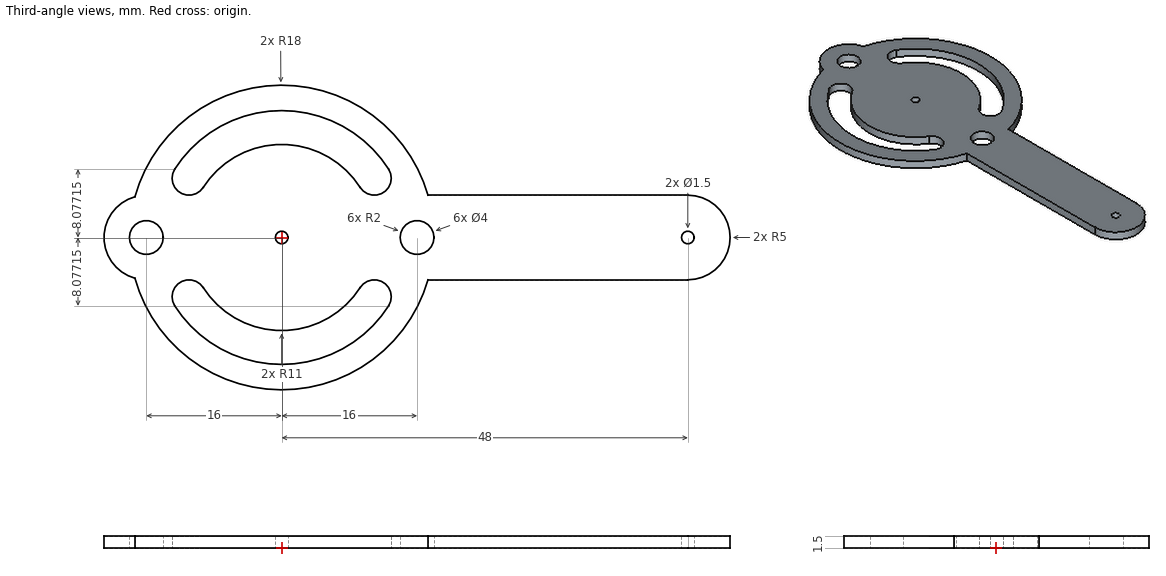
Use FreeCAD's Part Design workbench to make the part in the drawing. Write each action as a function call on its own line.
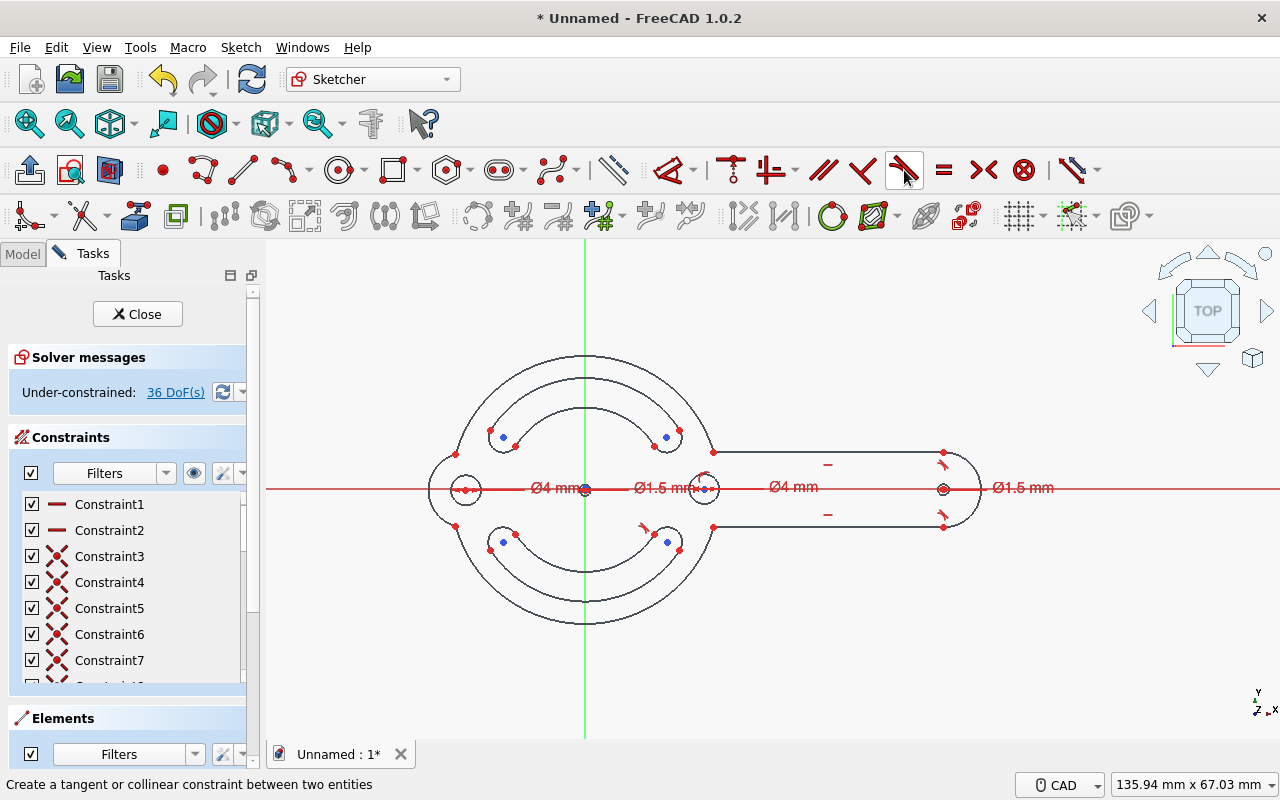
click(553, 565)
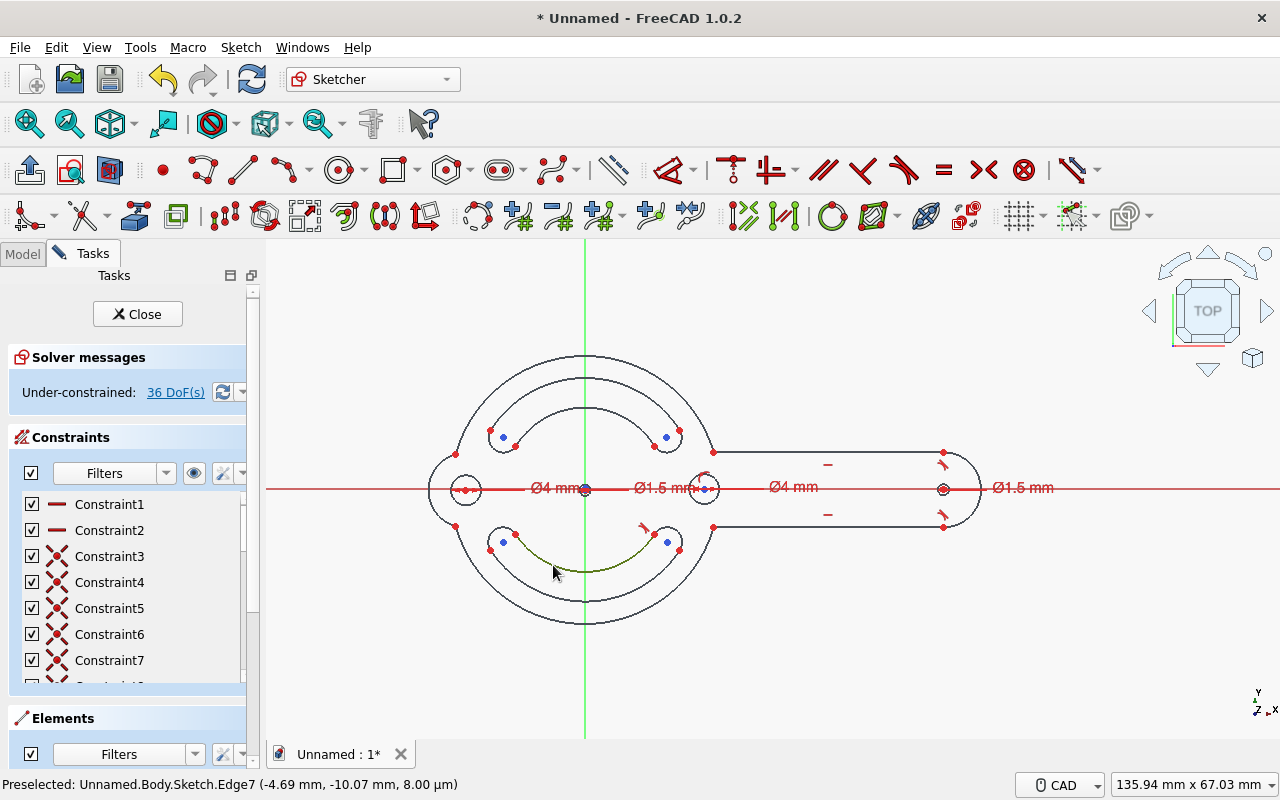
click(504, 527)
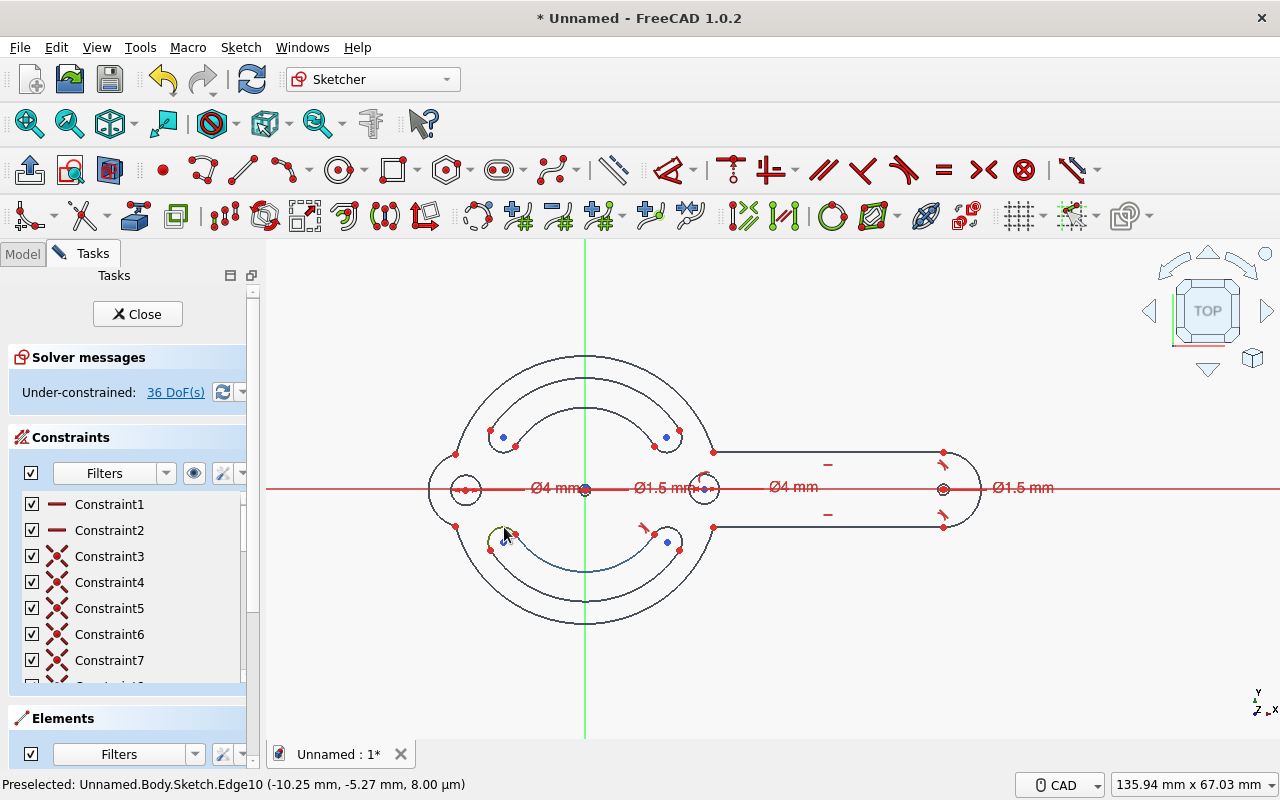
click(904, 170)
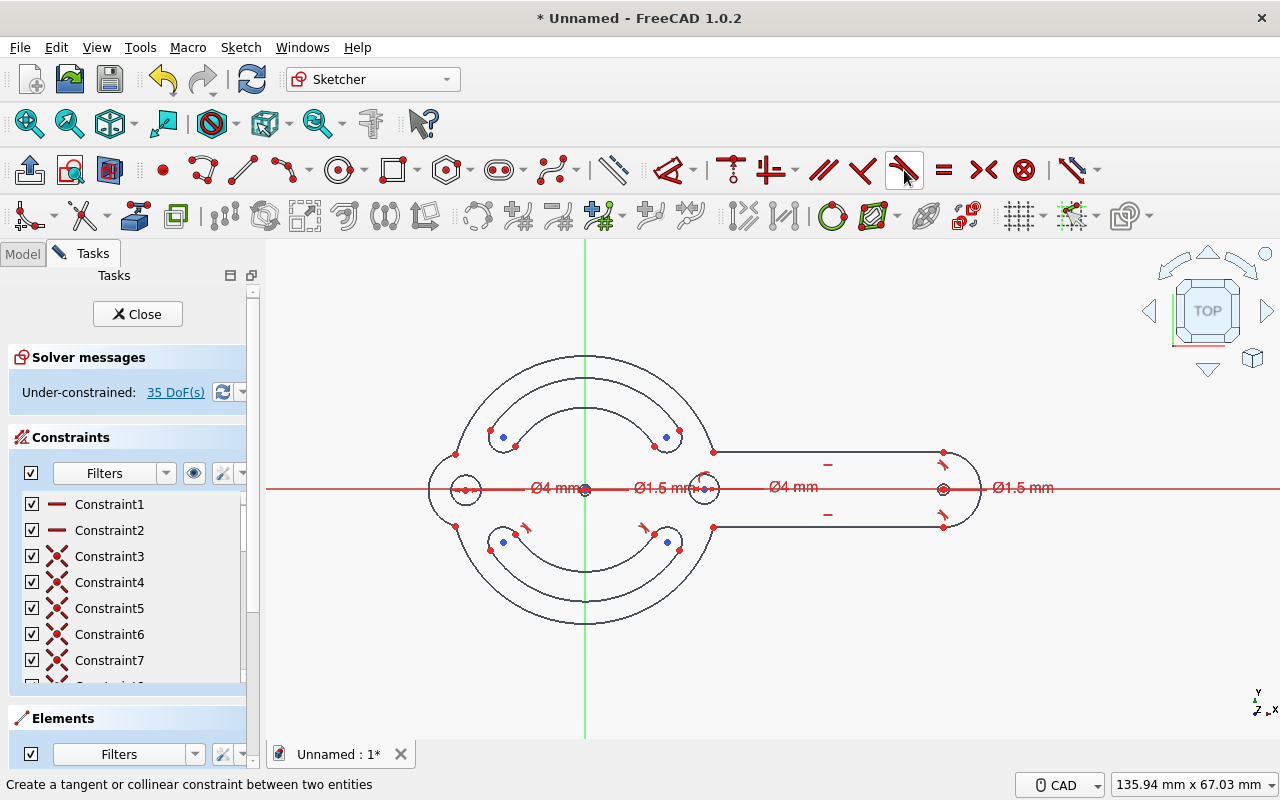
click(681, 537)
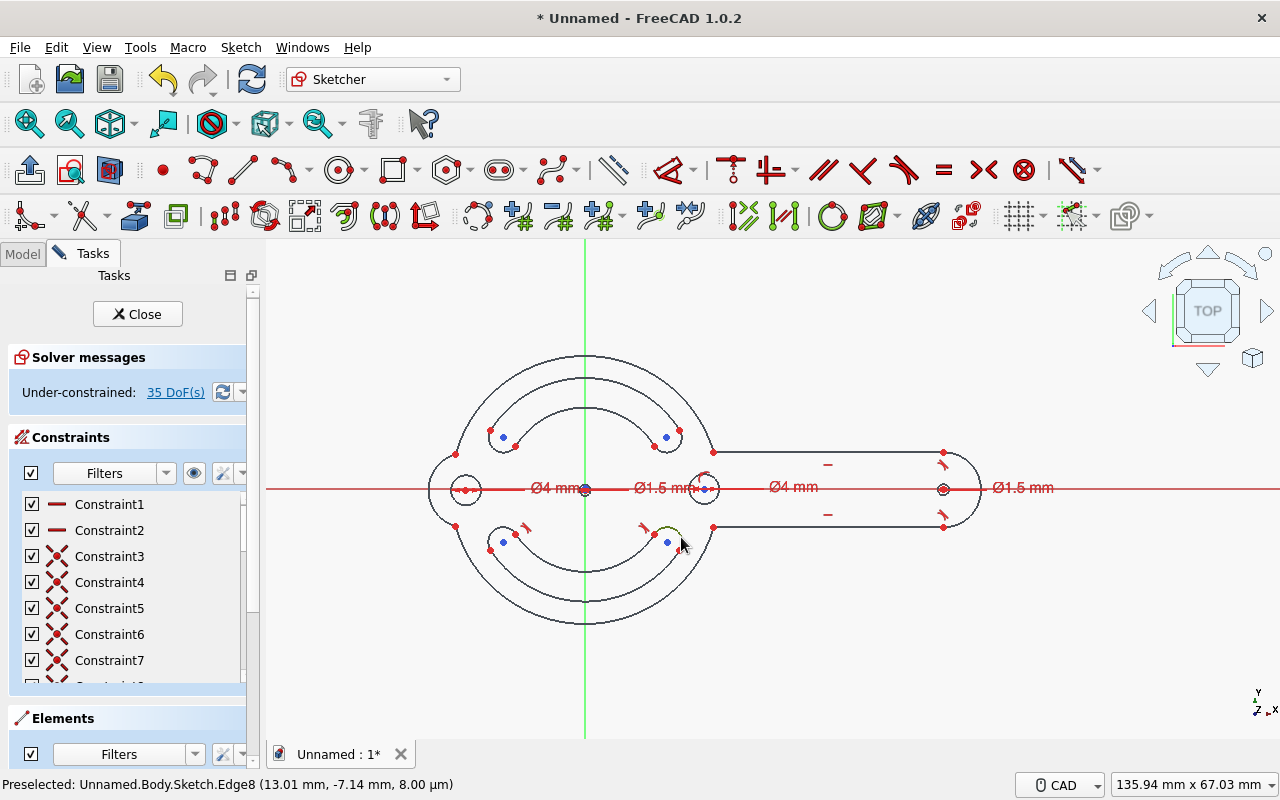
click(542, 593)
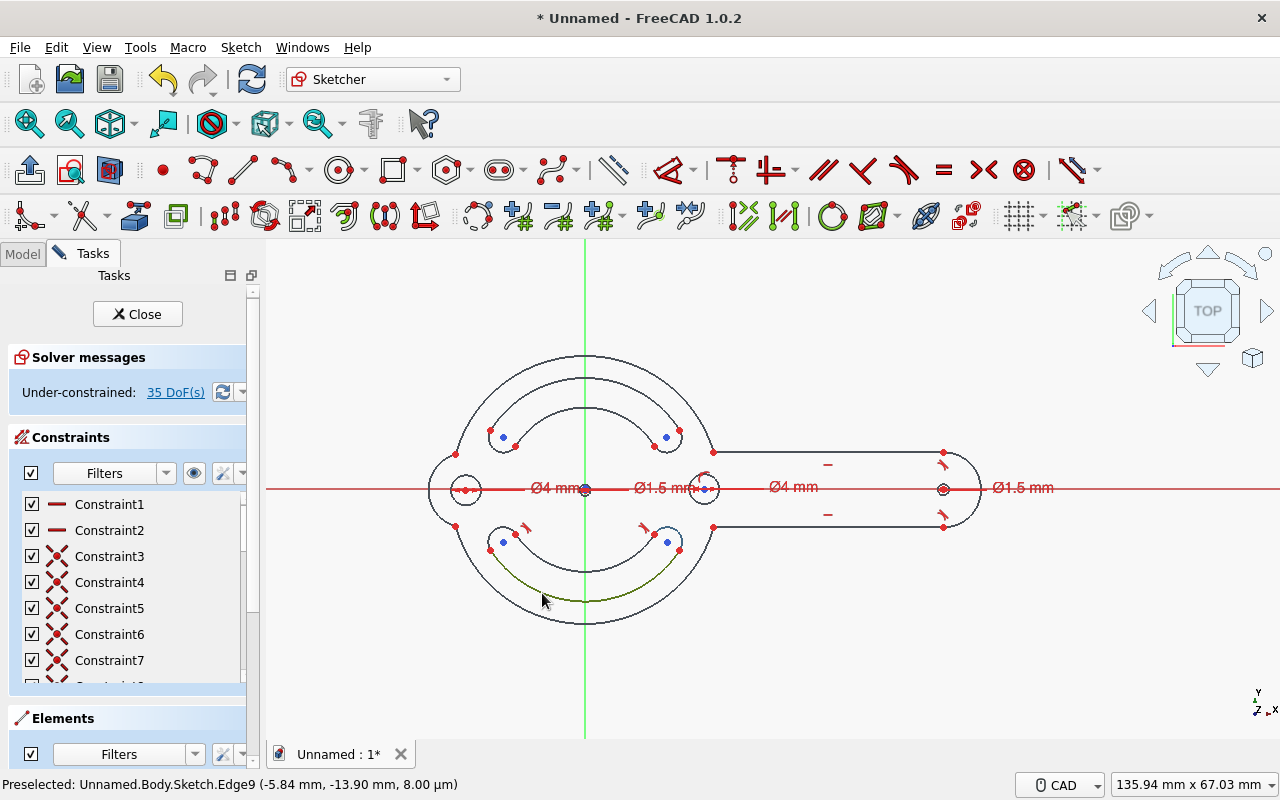
click(904, 170)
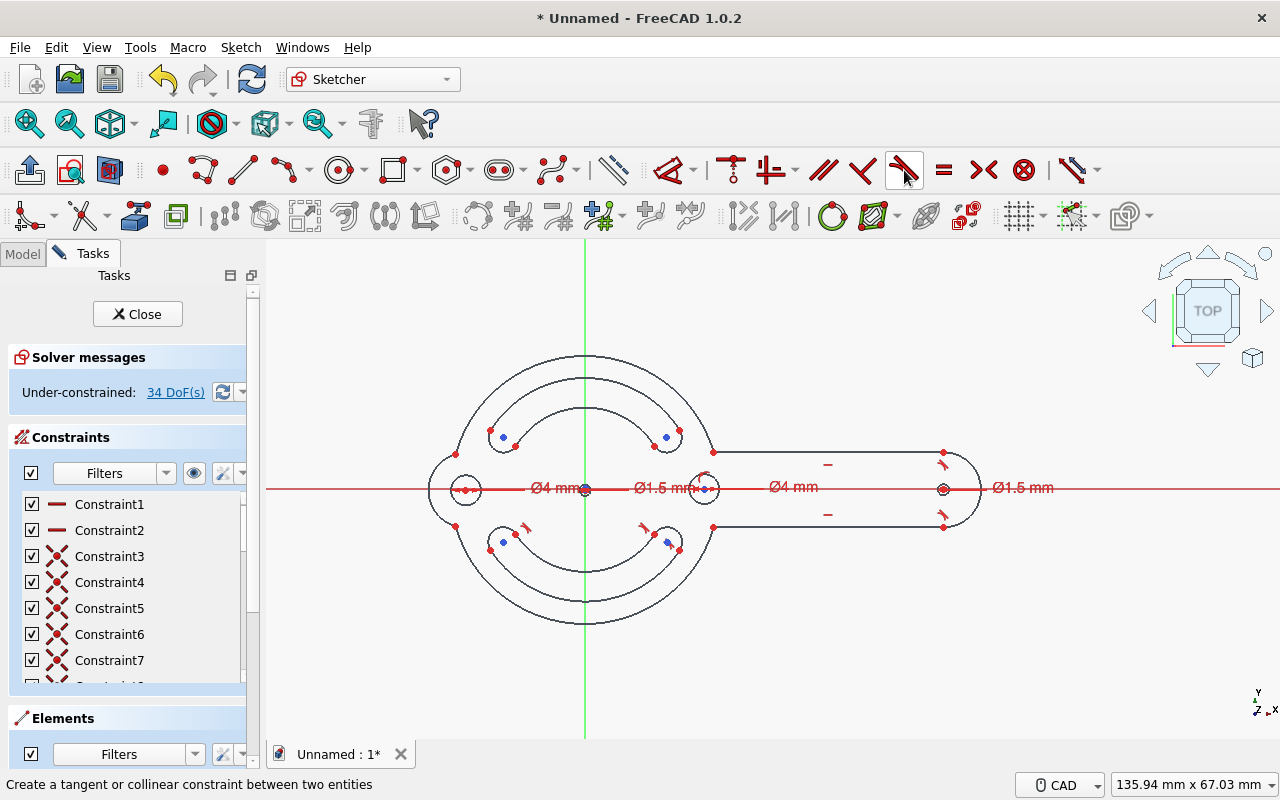
click(542, 593)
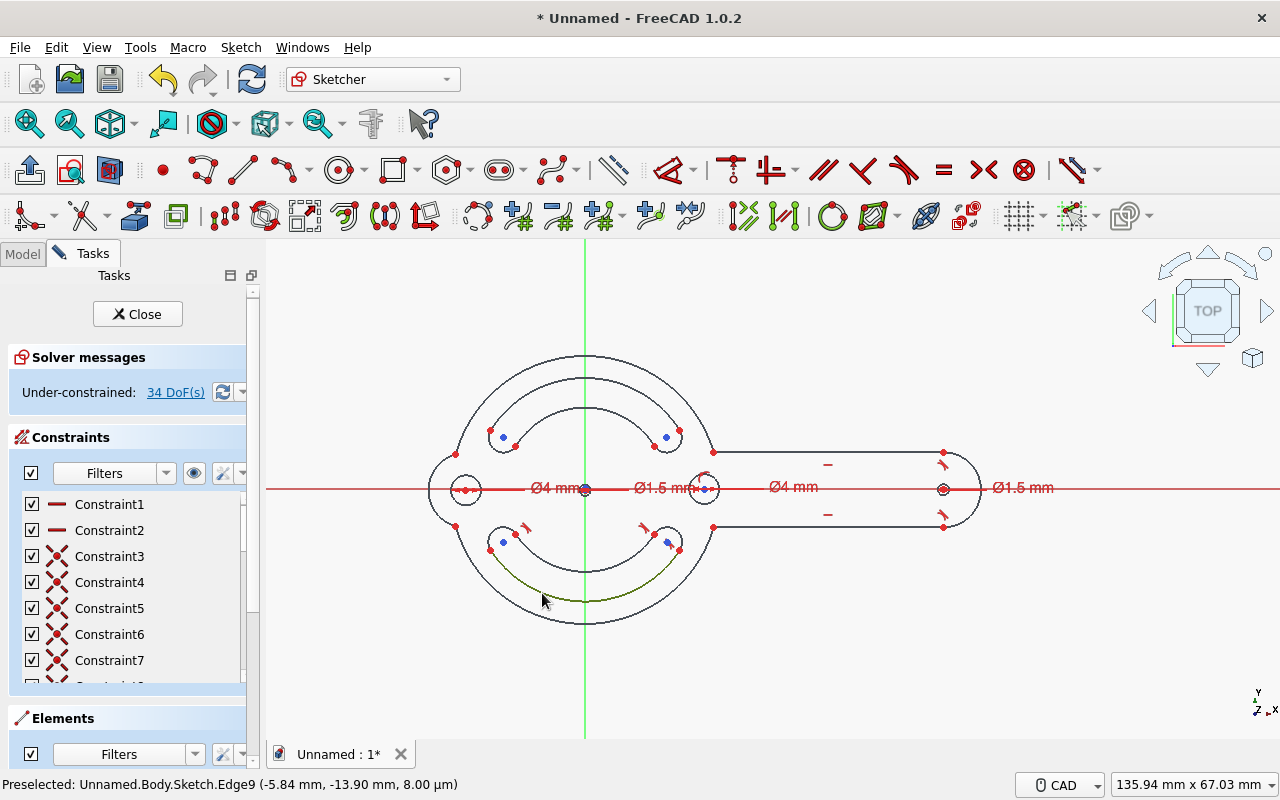
click(504, 527)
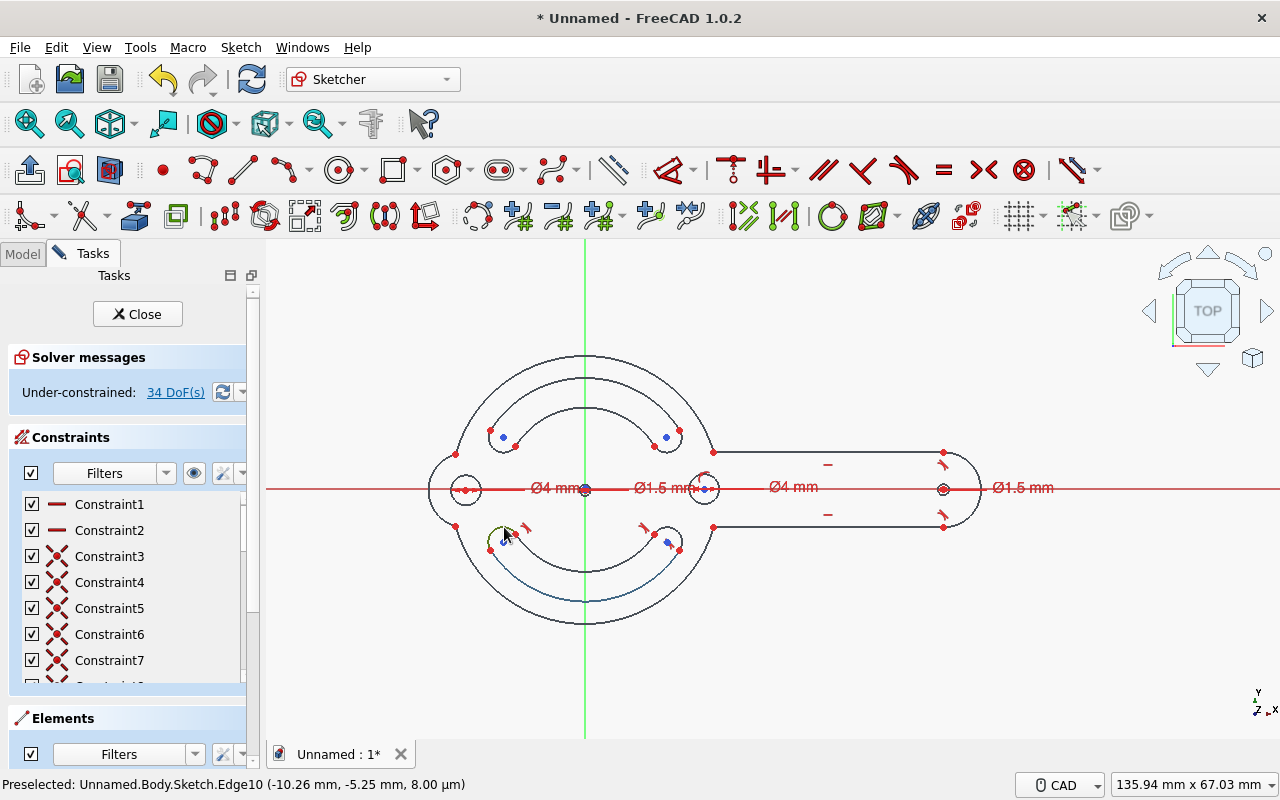
click(904, 170)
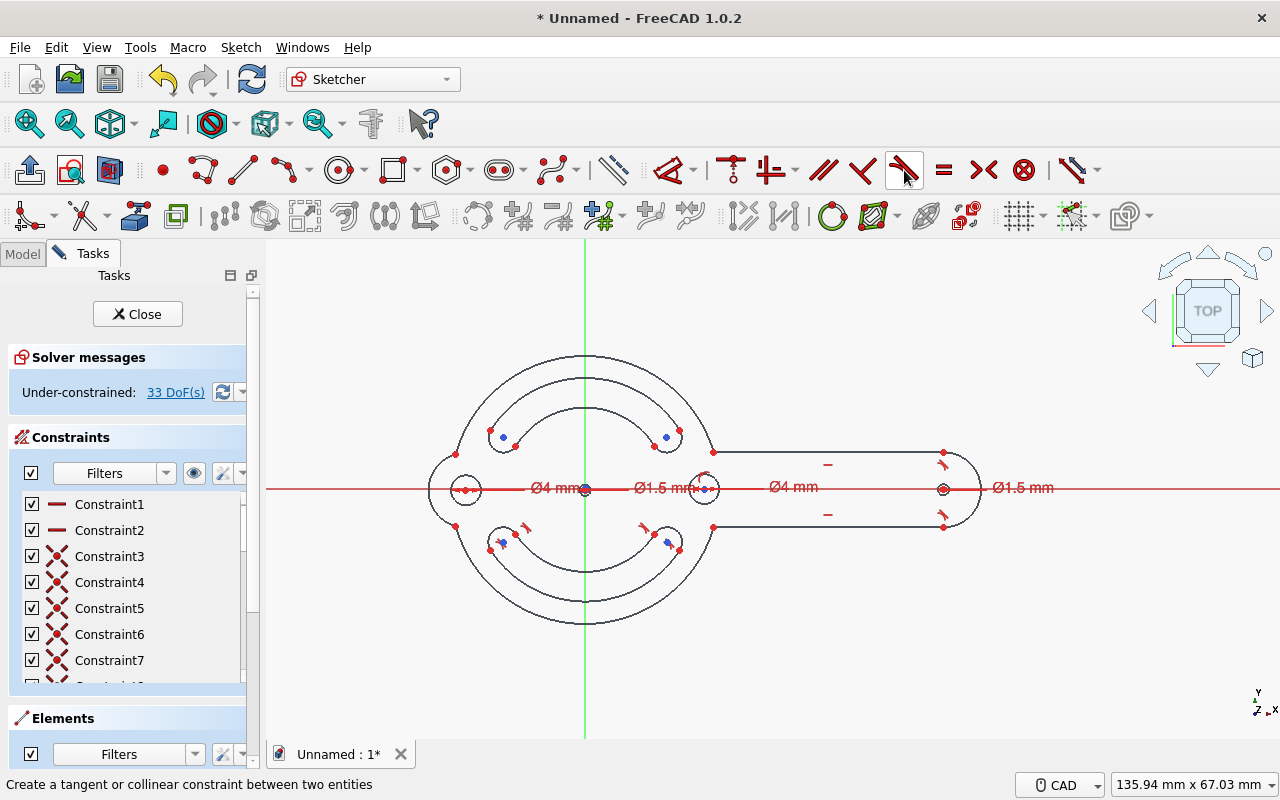
click(618, 414)